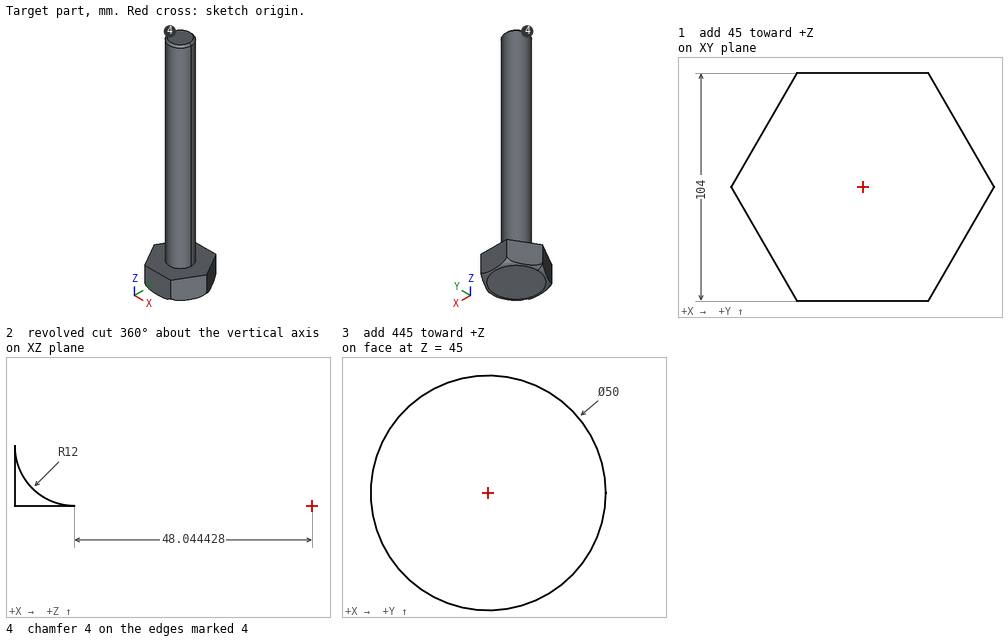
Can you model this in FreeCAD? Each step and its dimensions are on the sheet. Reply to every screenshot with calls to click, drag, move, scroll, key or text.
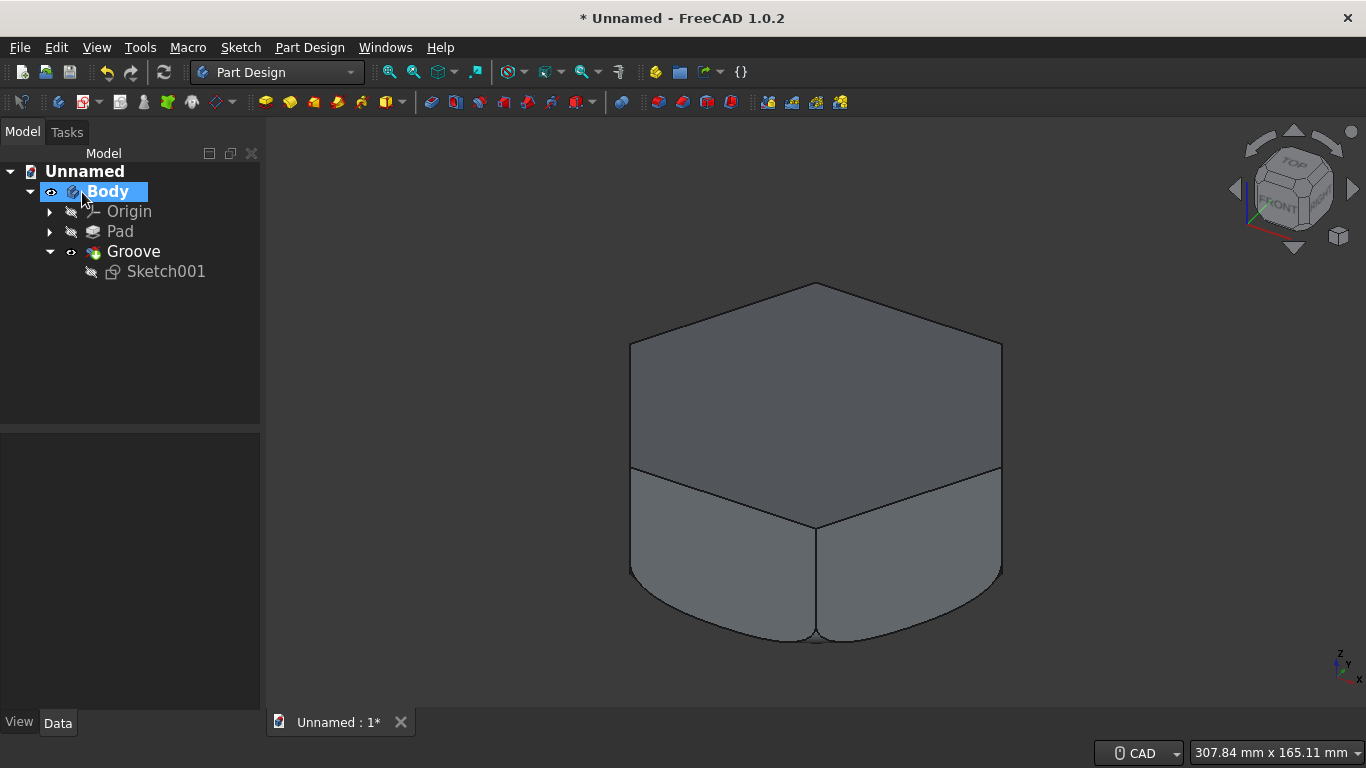
click(816, 405)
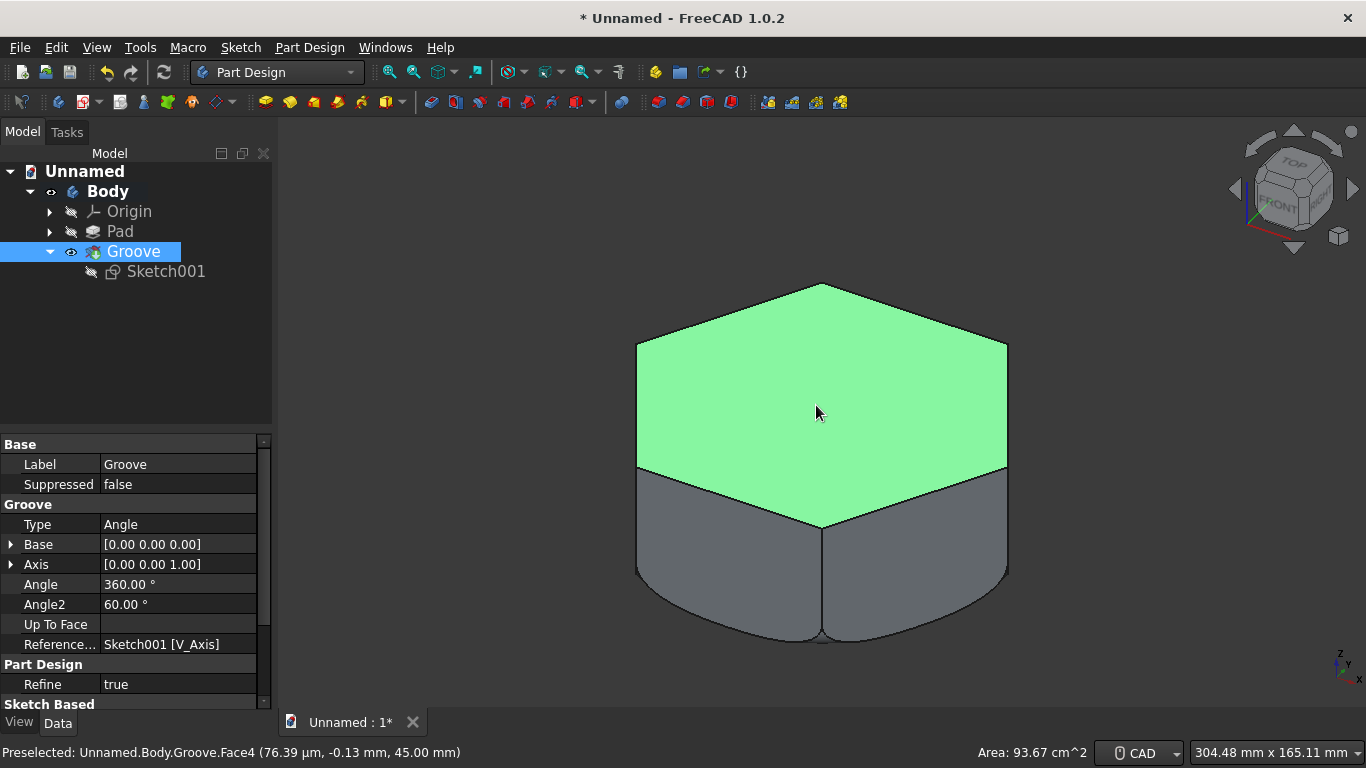
click(84, 102)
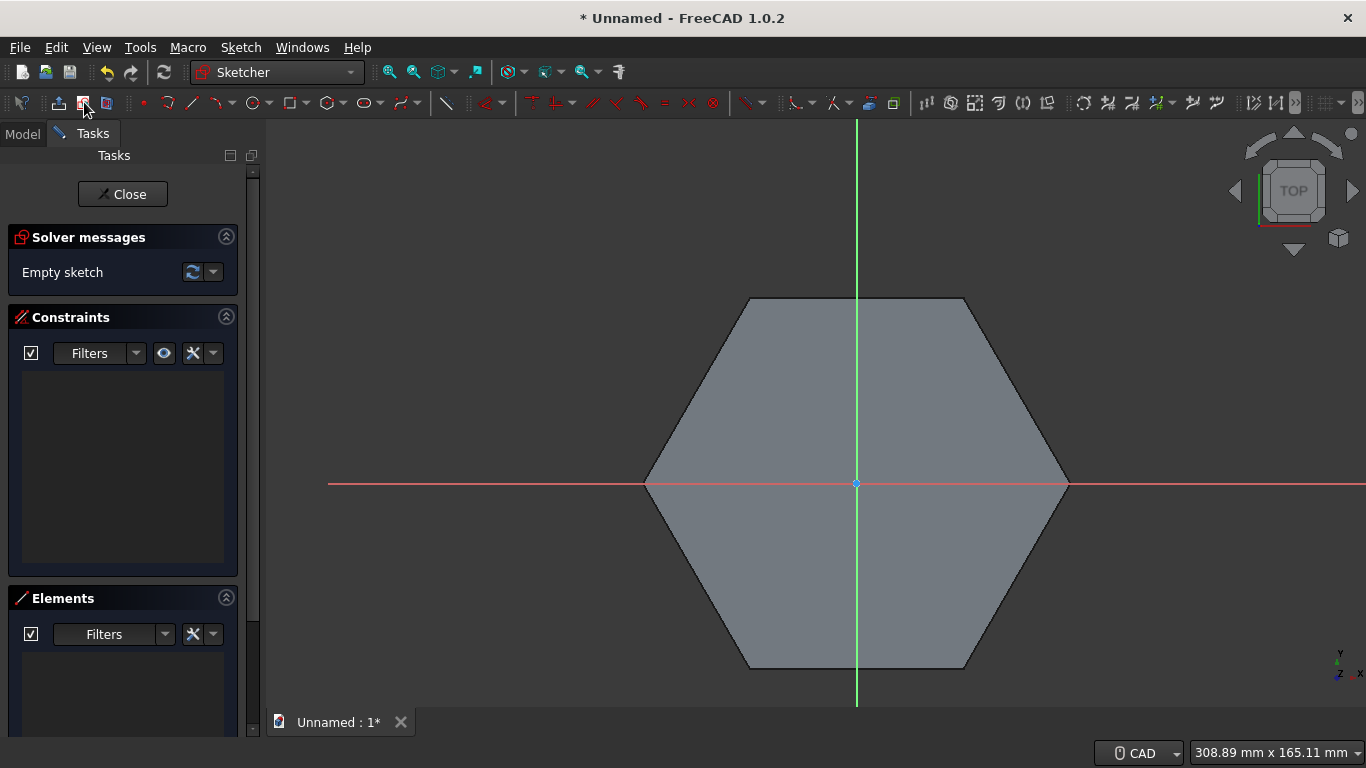
scroll(946, 541, up, 4)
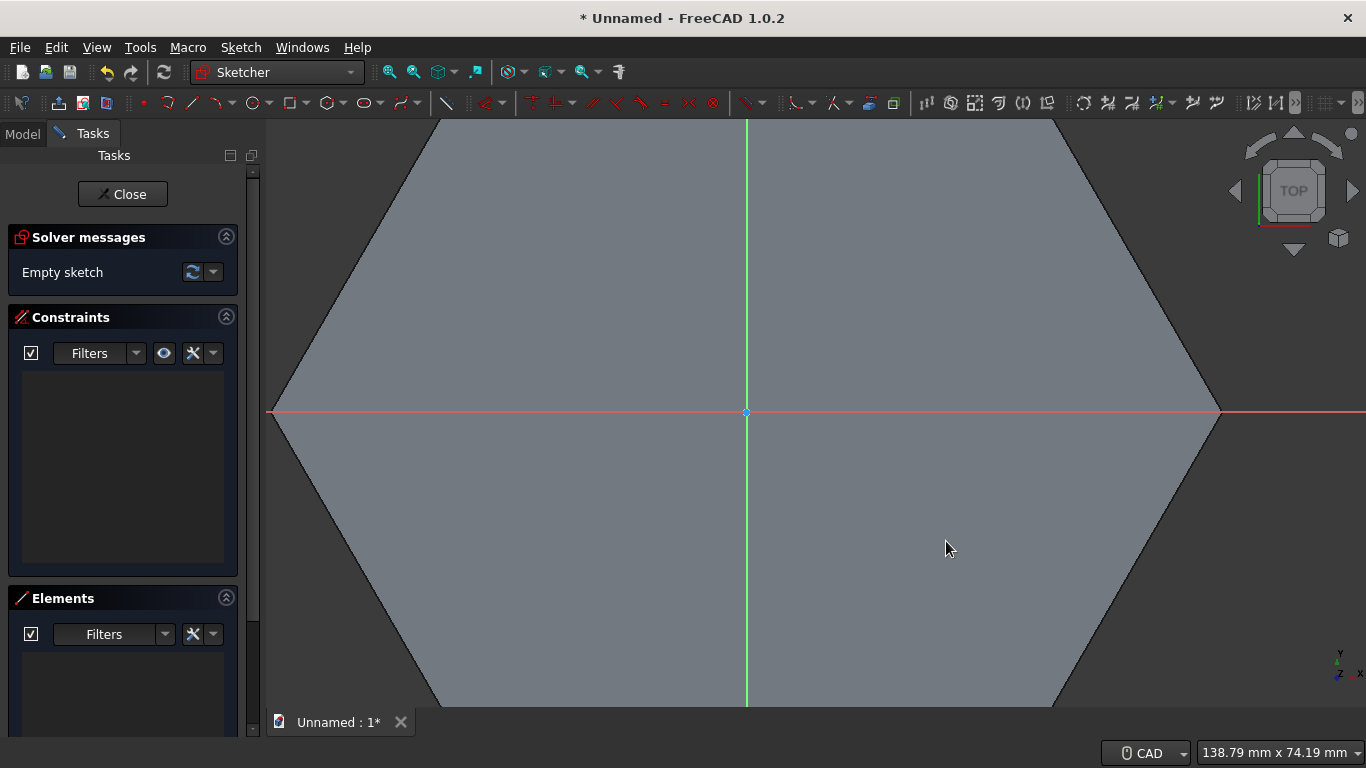
key(g)
key(c)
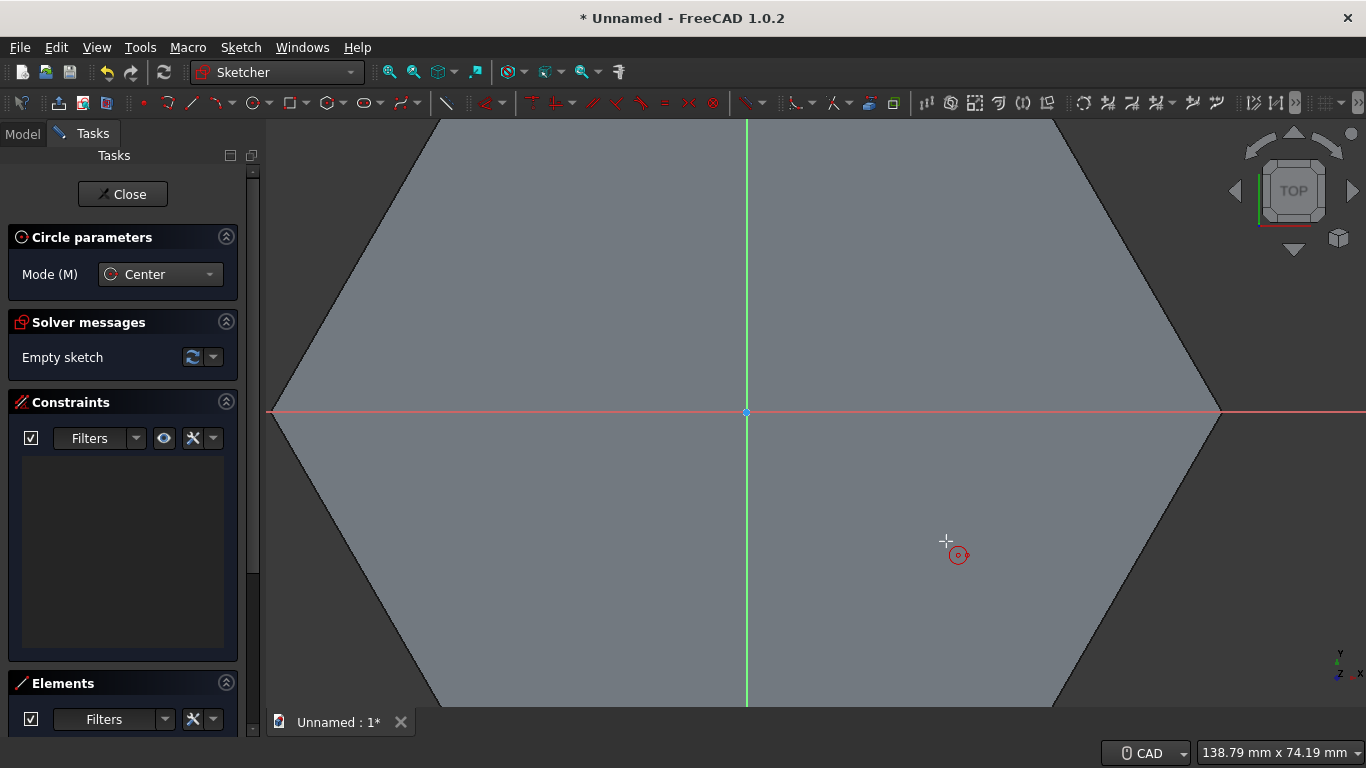
click(747, 412)
click(887, 272)
key(Escape)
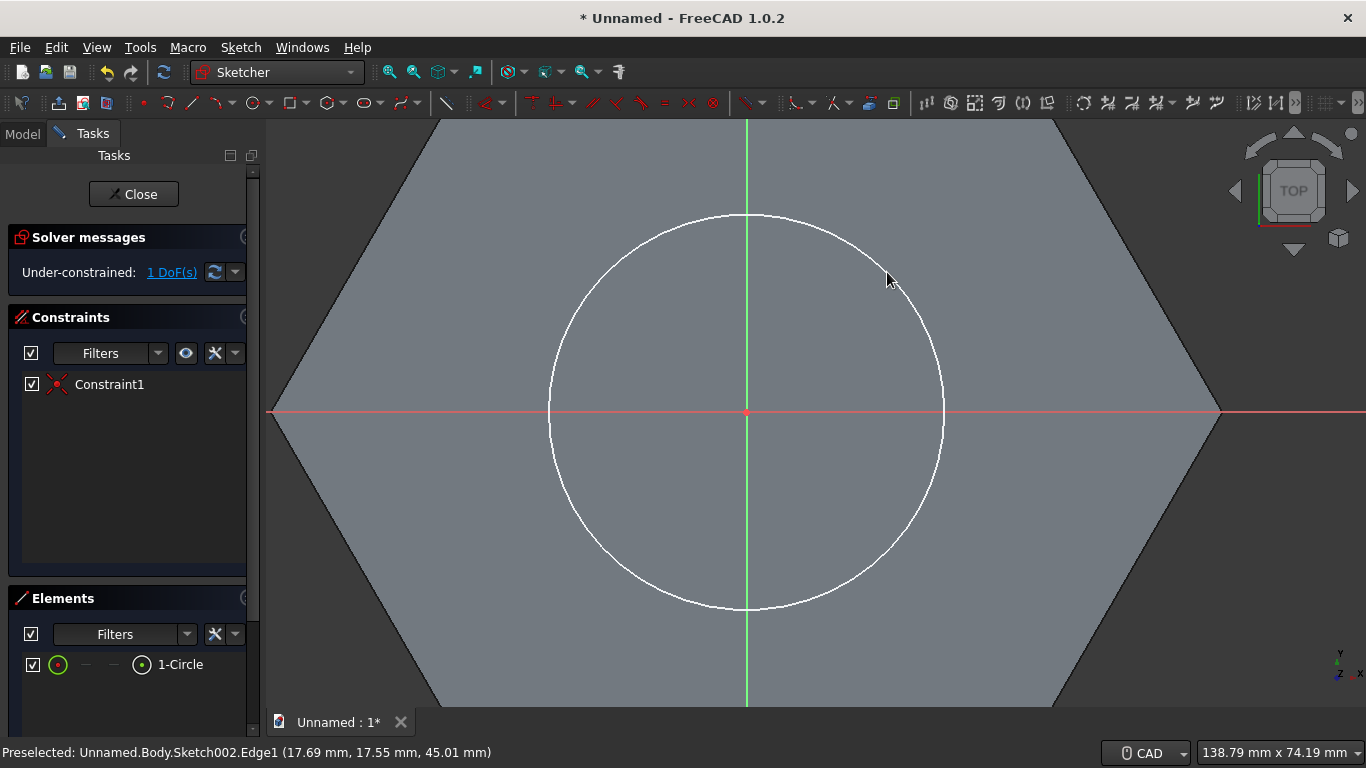
click(486, 104)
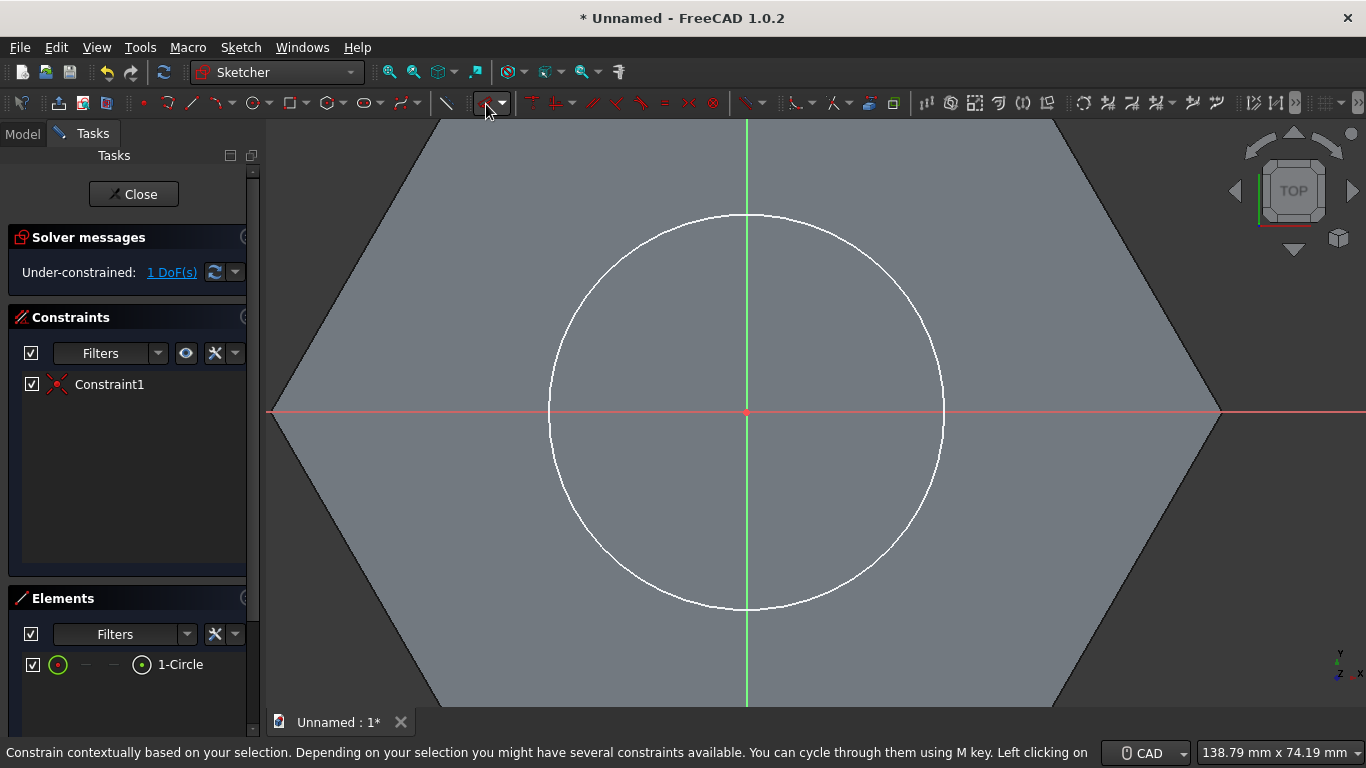
click(886, 272)
click(909, 249)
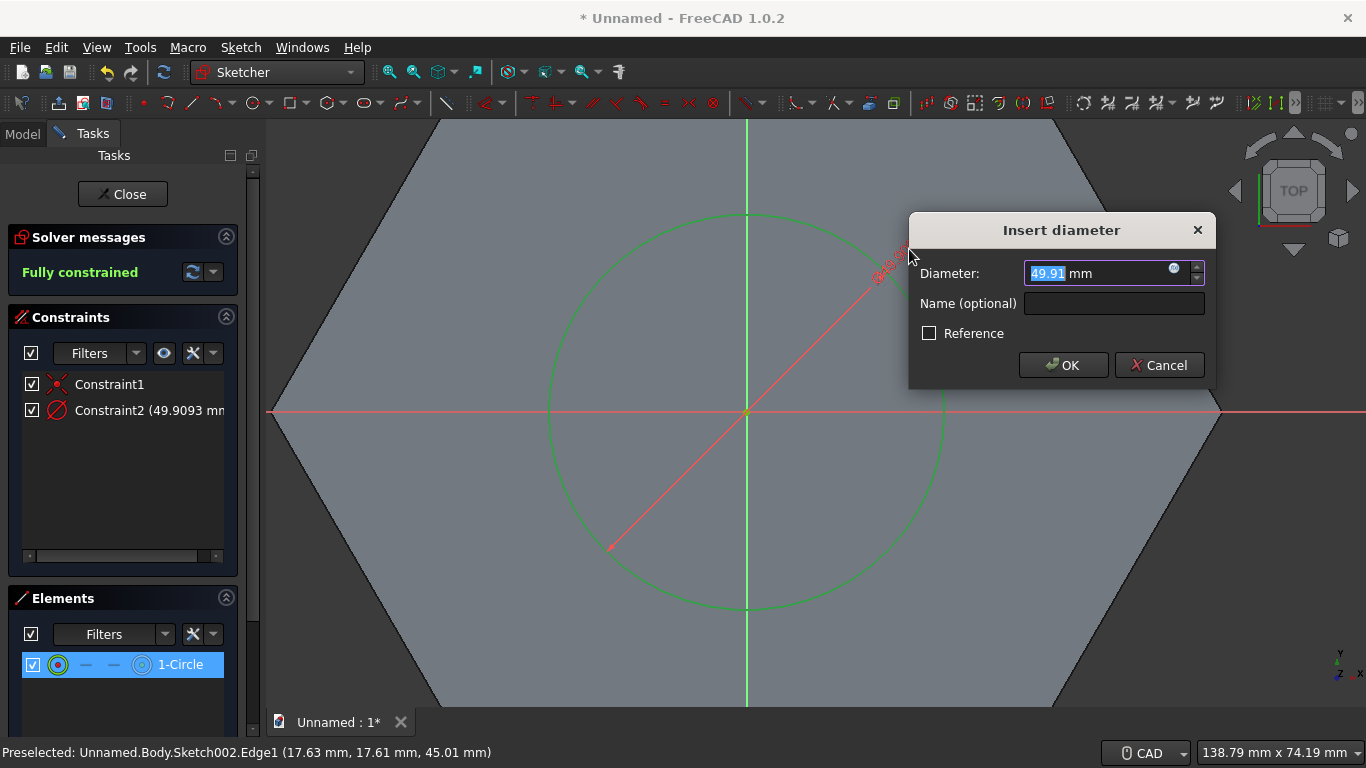
text(50)
key(Return)
key(Escape)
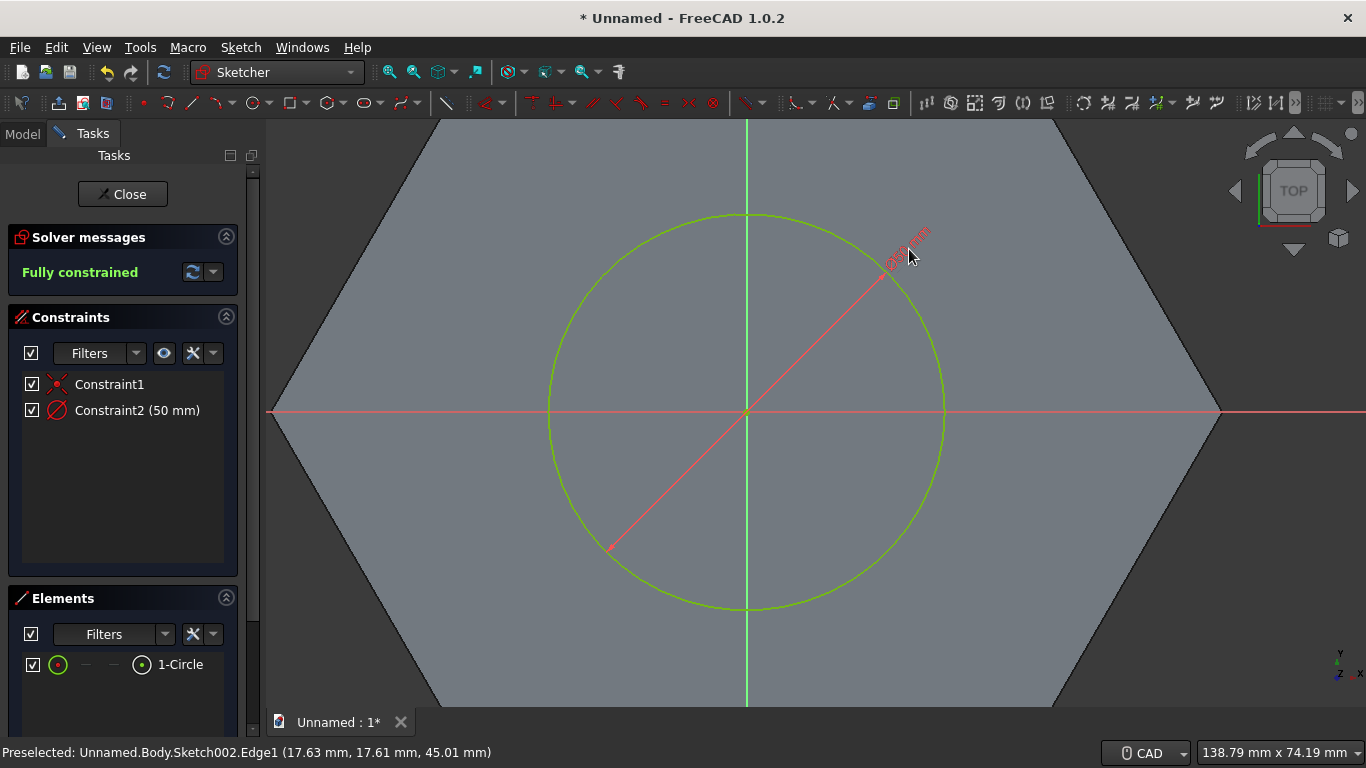
click(123, 194)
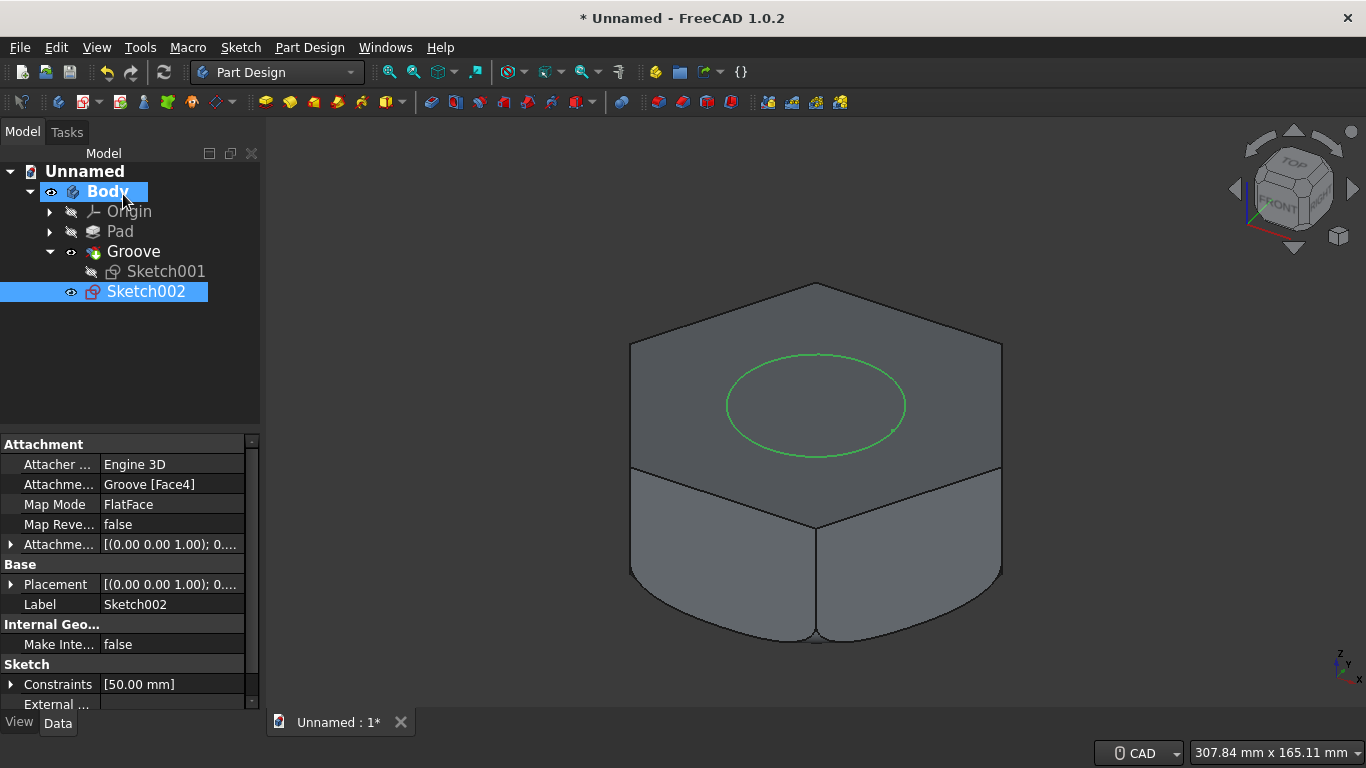
click(266, 102)